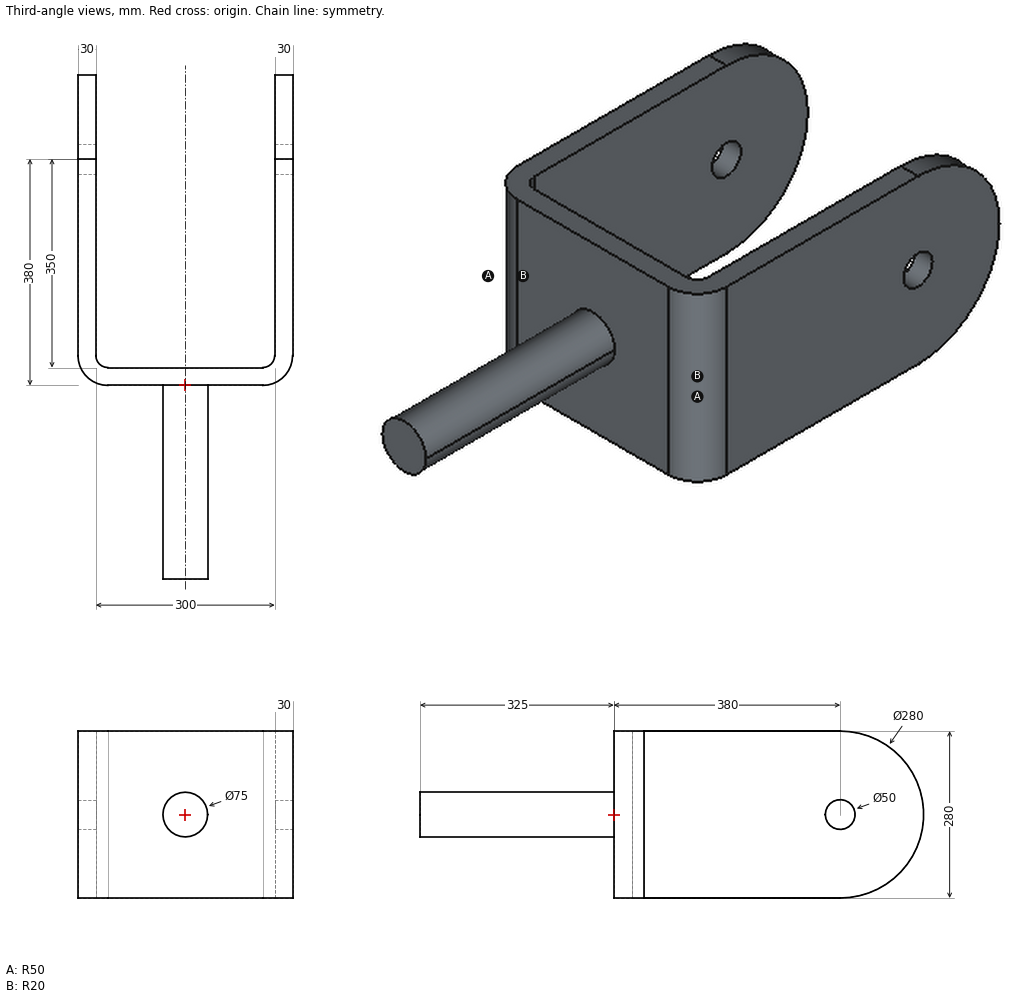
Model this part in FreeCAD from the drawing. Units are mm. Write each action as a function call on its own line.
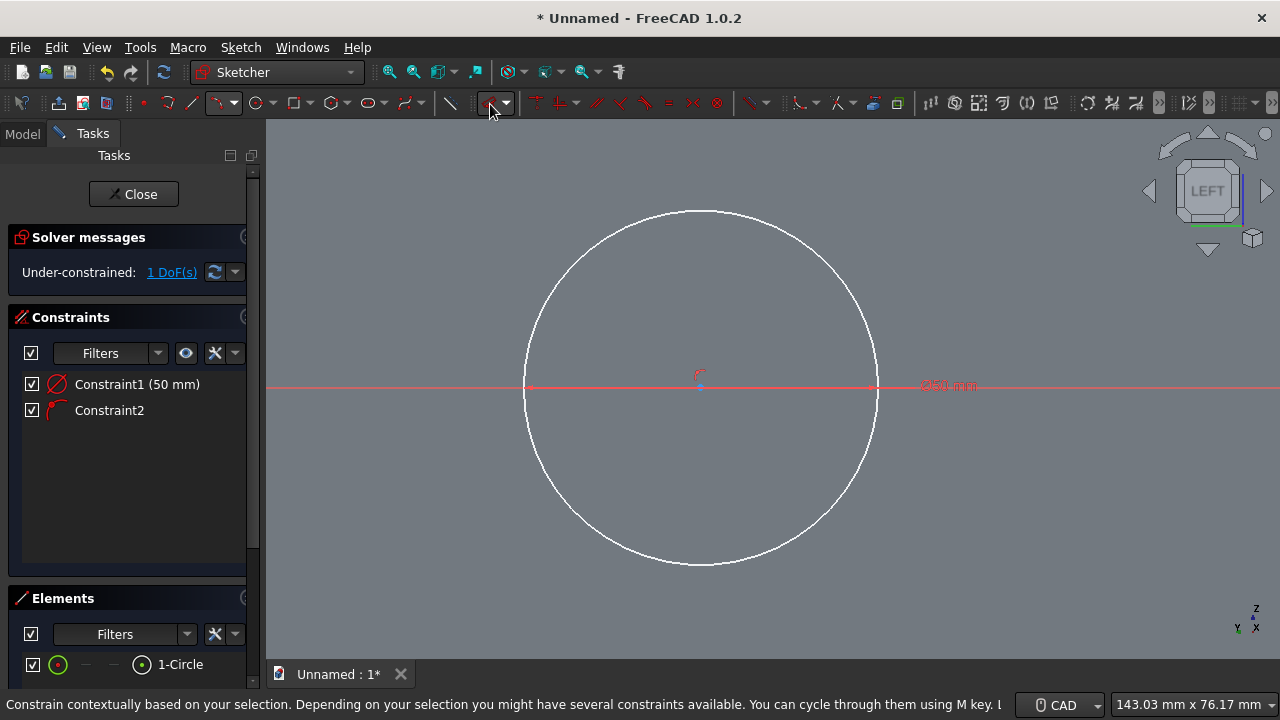
click(701, 388)
click(908, 422)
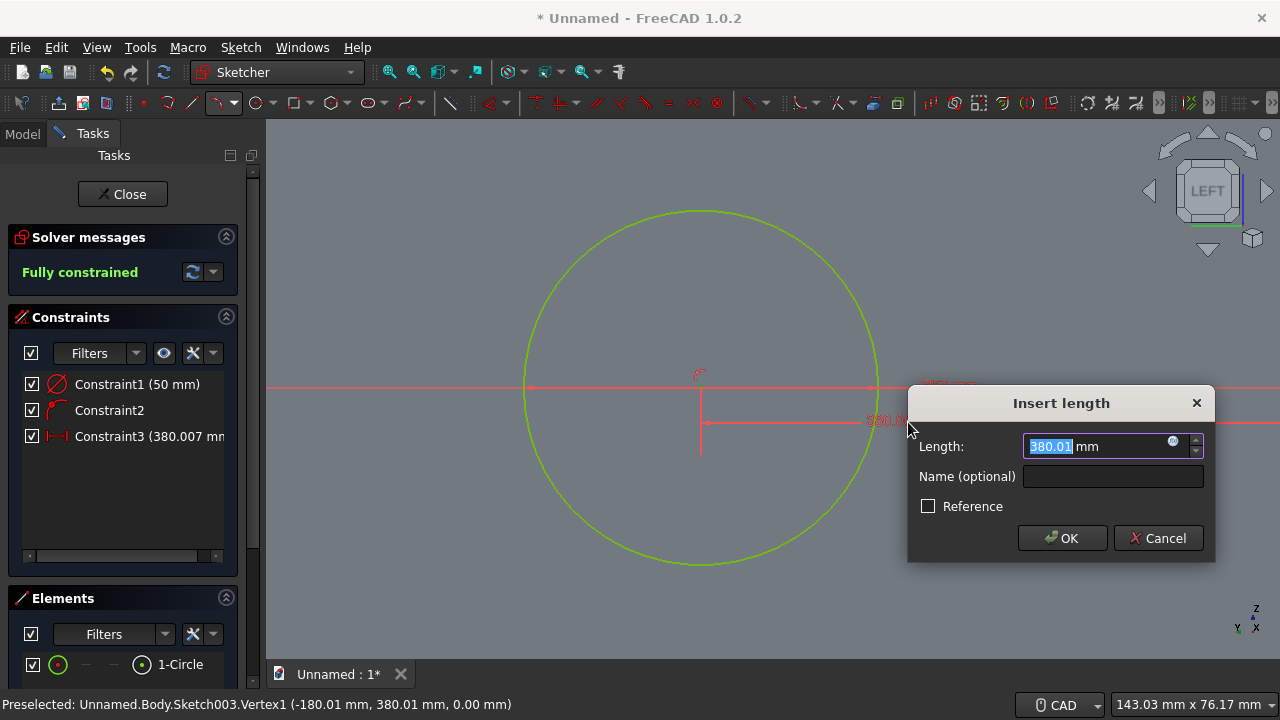
text(380)
key(Return)
key(Escape)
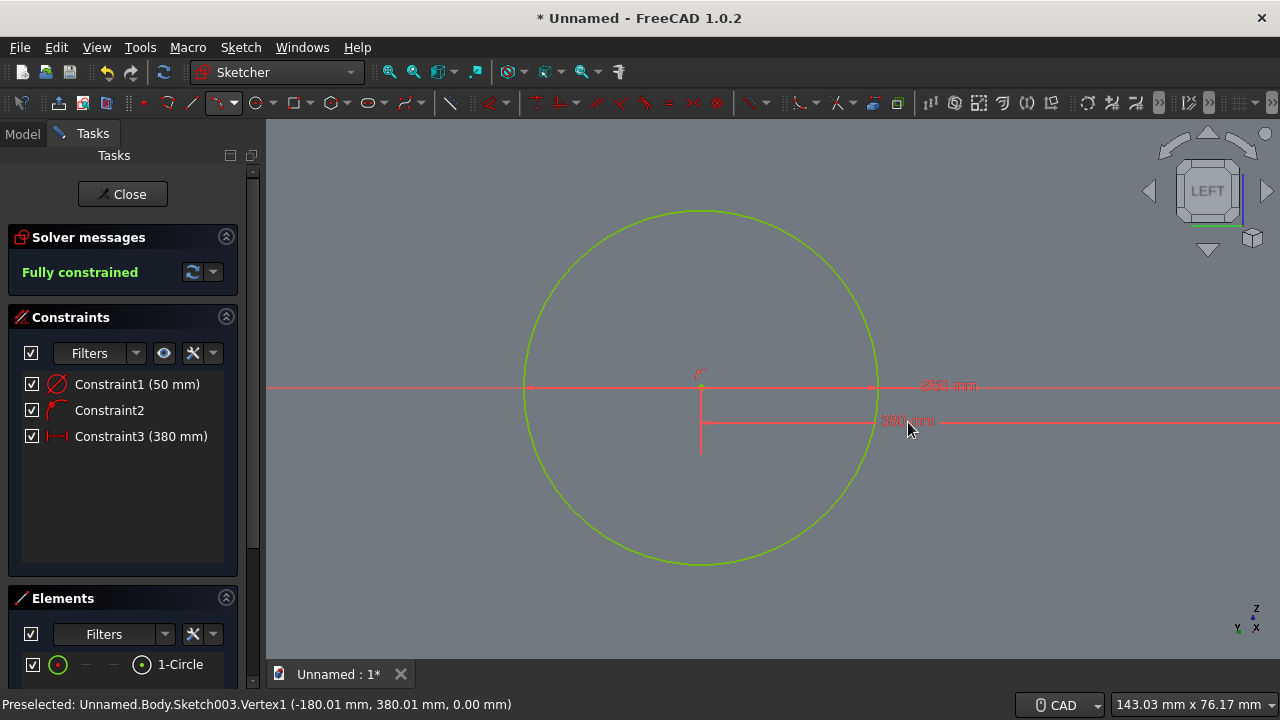
click(123, 194)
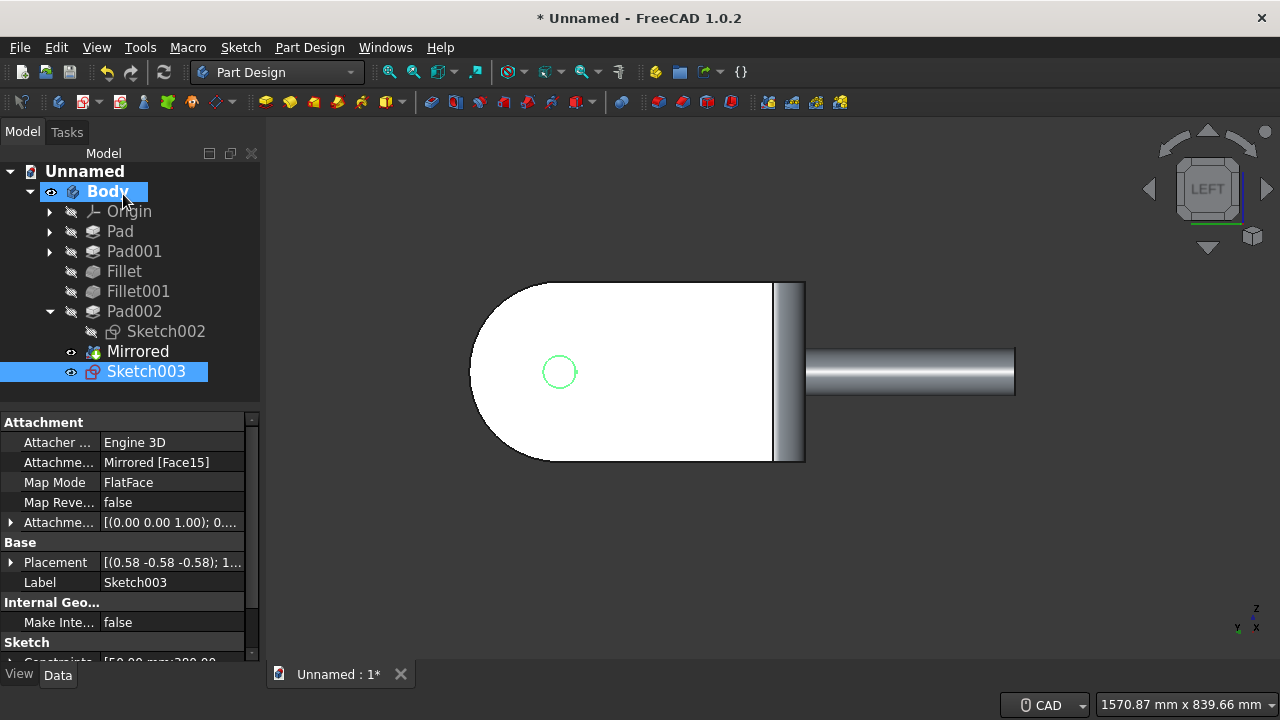
click(432, 102)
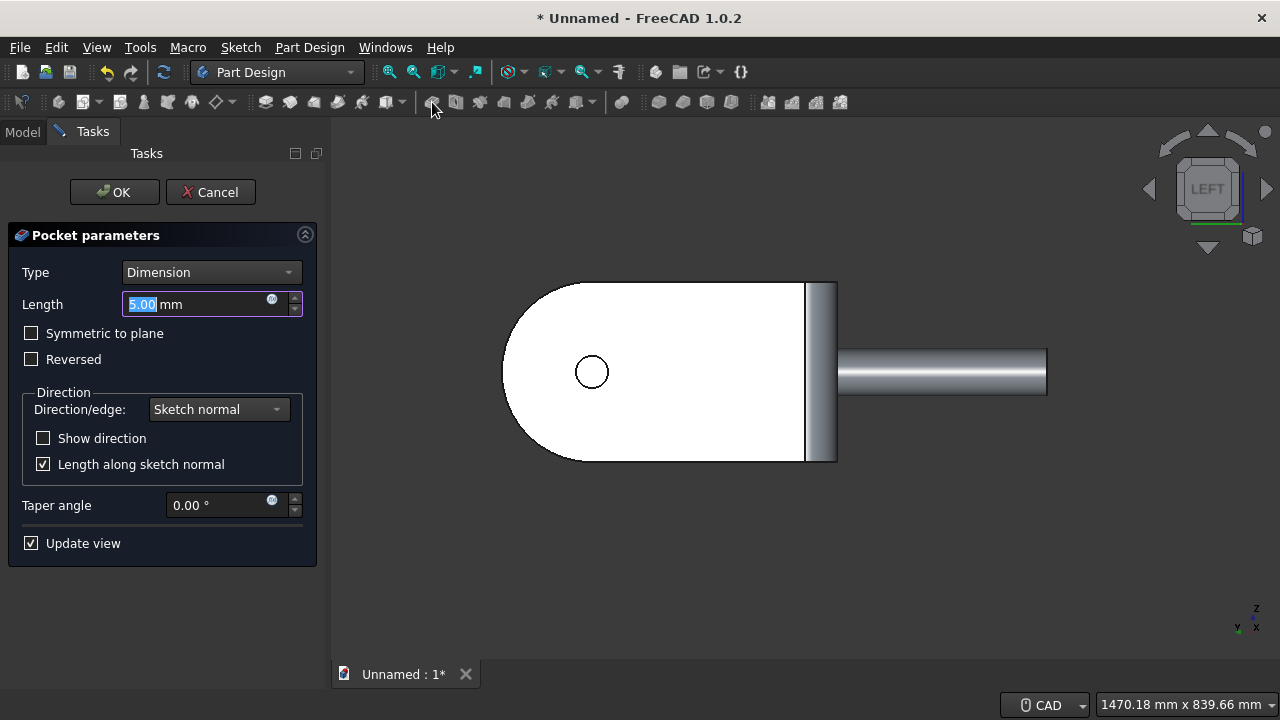
click(212, 272)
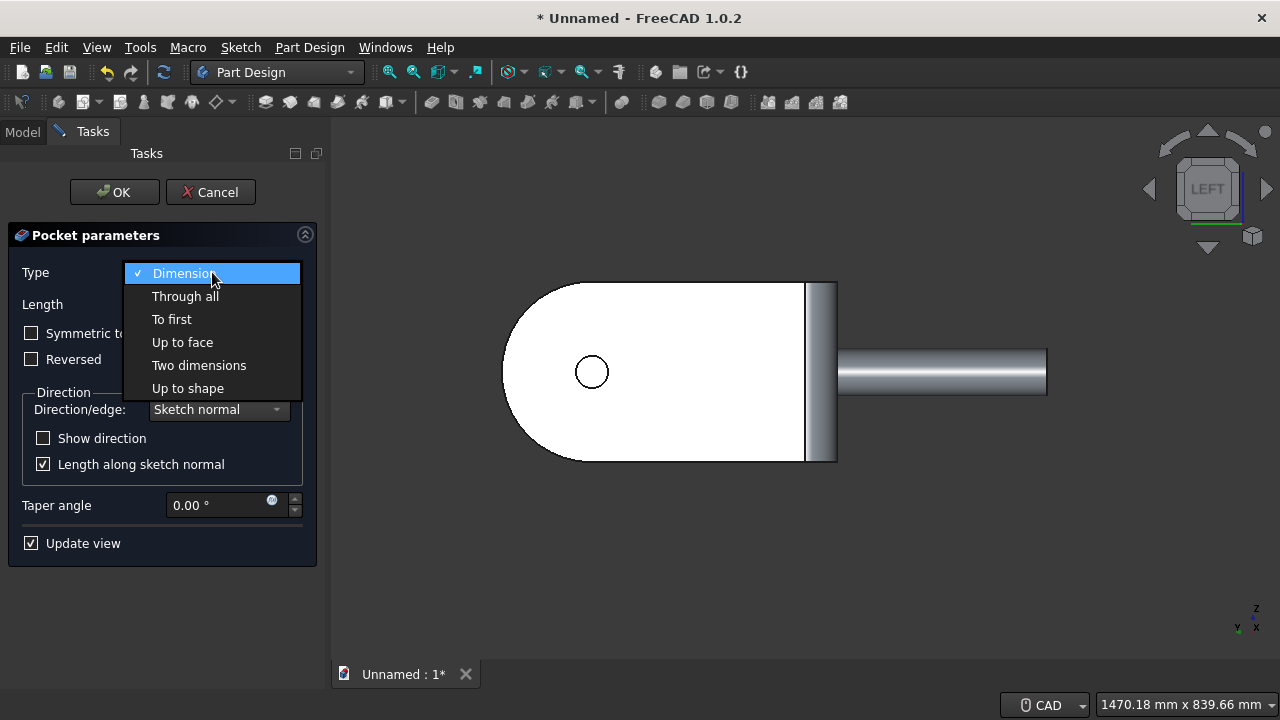
click(212, 296)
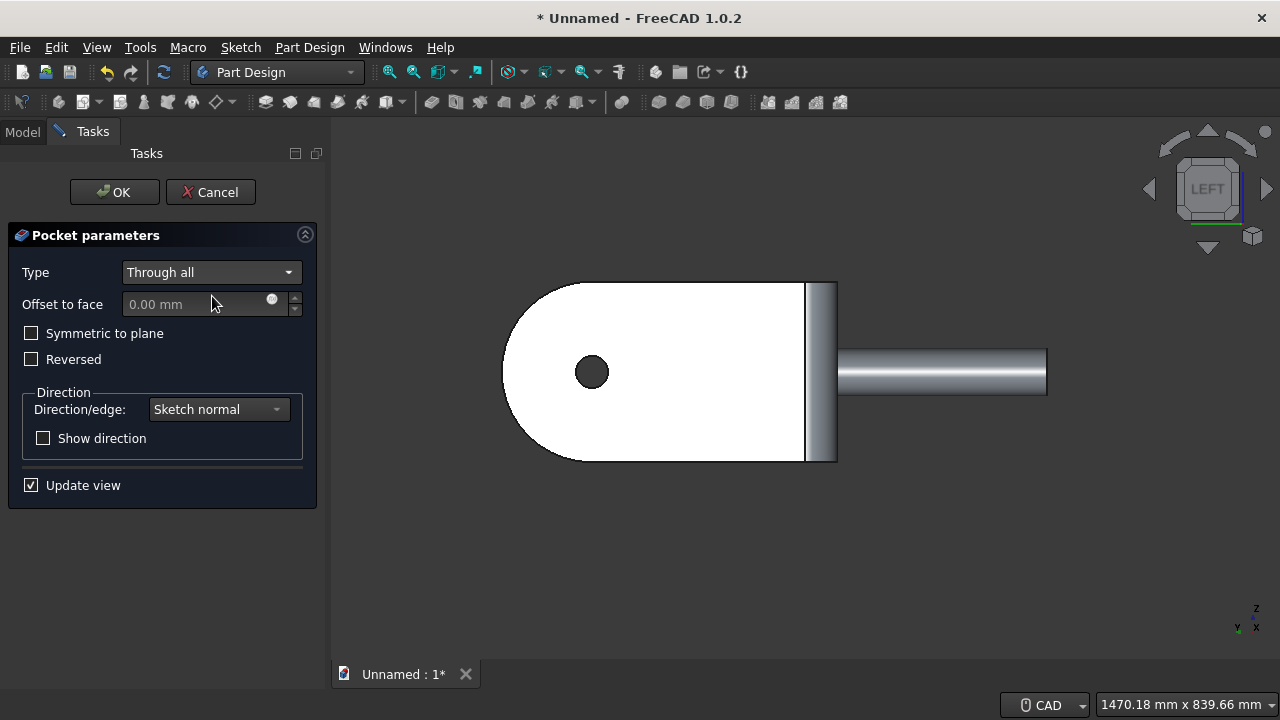
click(115, 192)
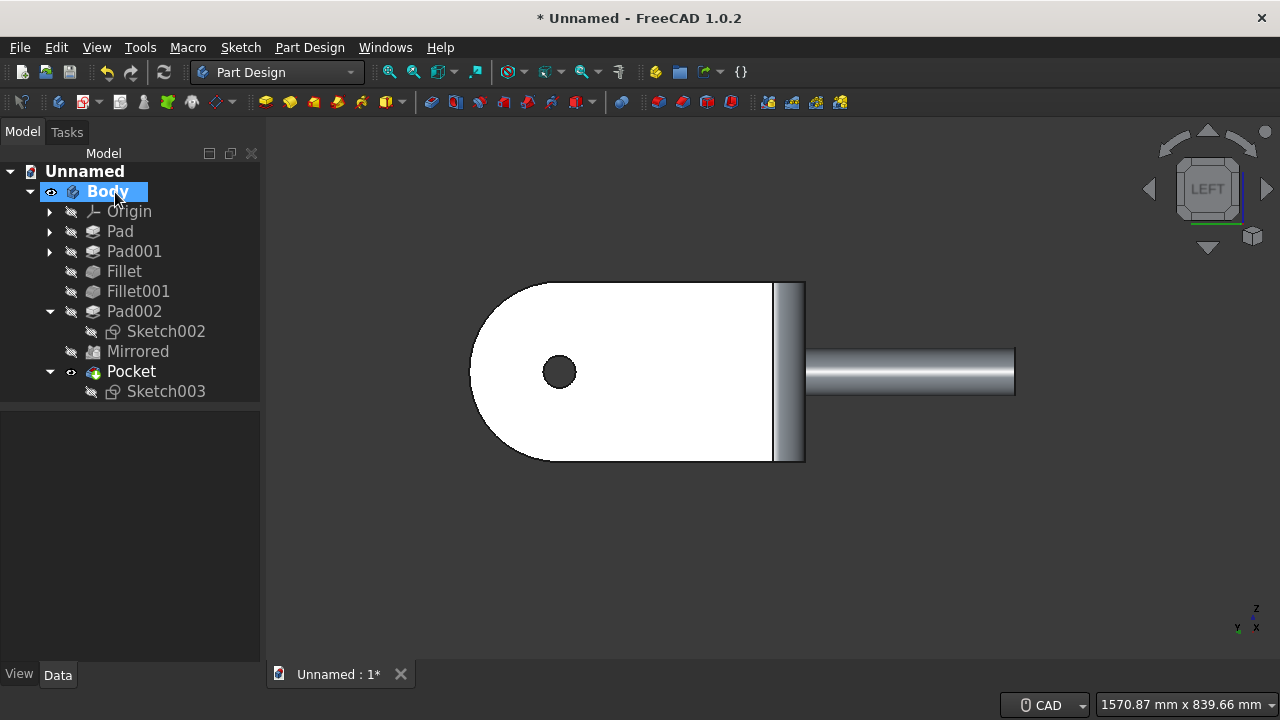
key(0)